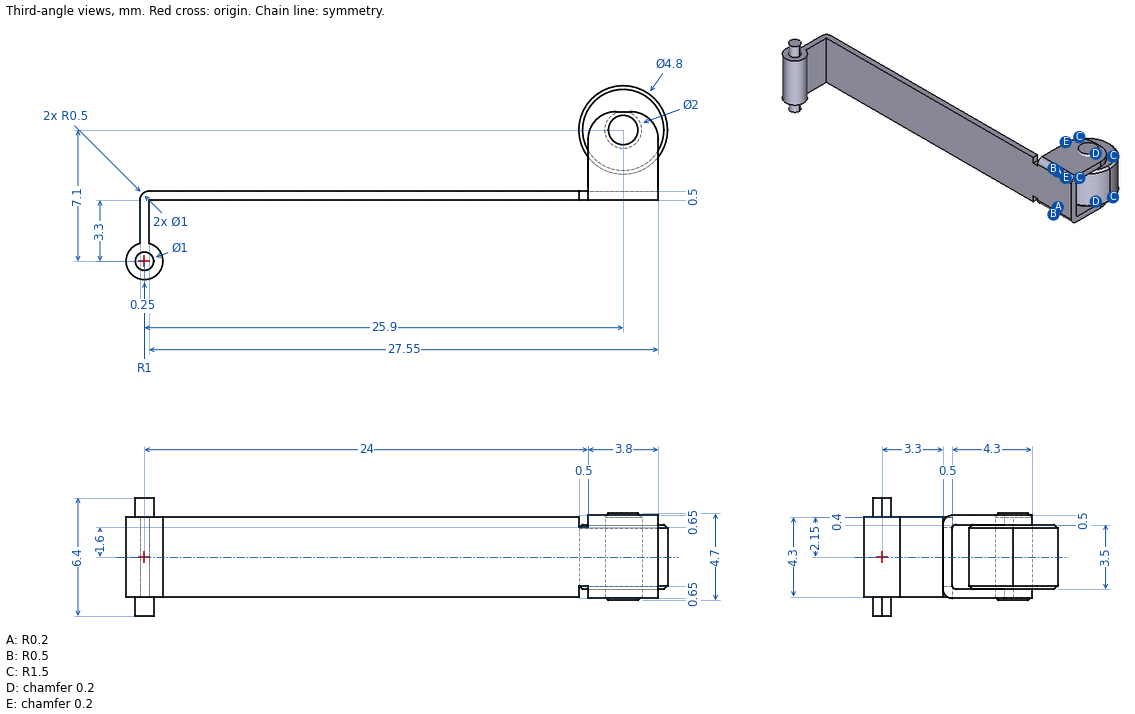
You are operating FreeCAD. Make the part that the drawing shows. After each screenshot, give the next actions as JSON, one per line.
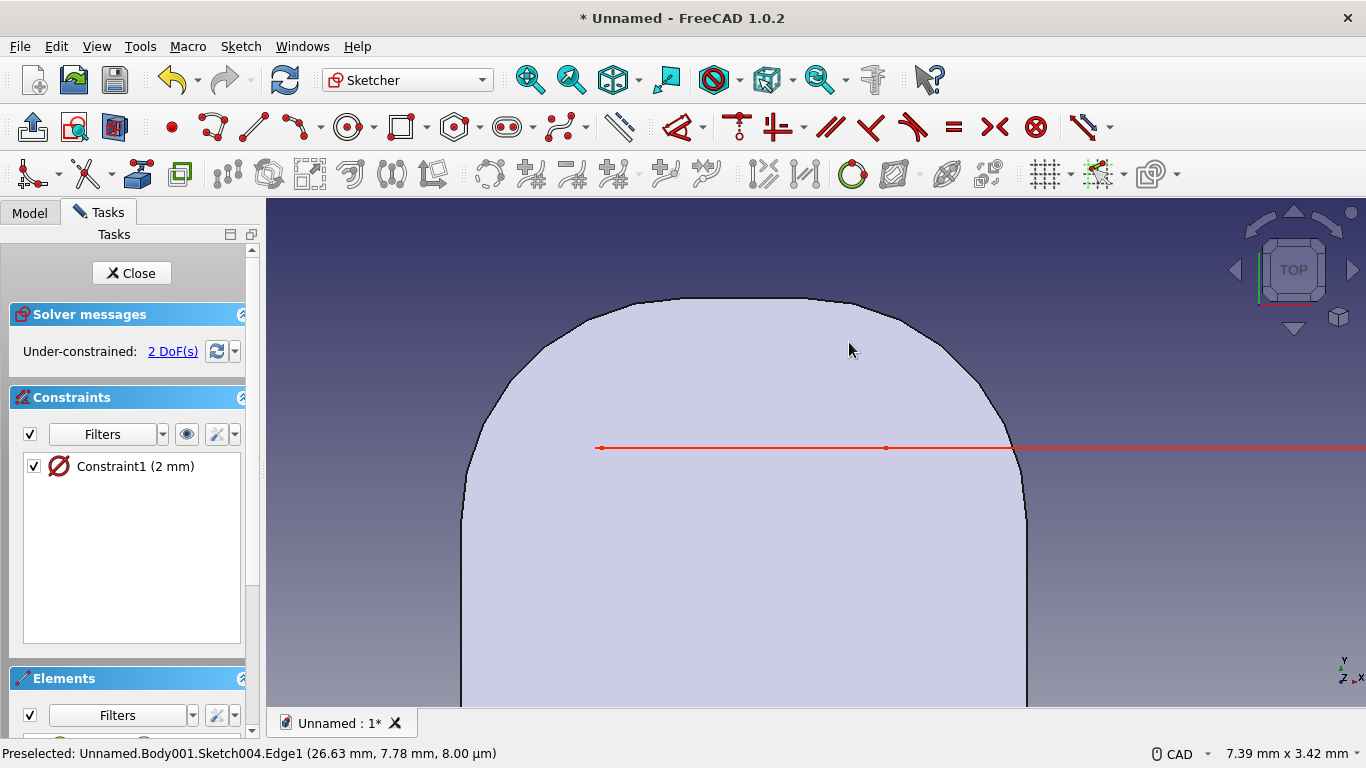
{"action": "key", "text": "d"}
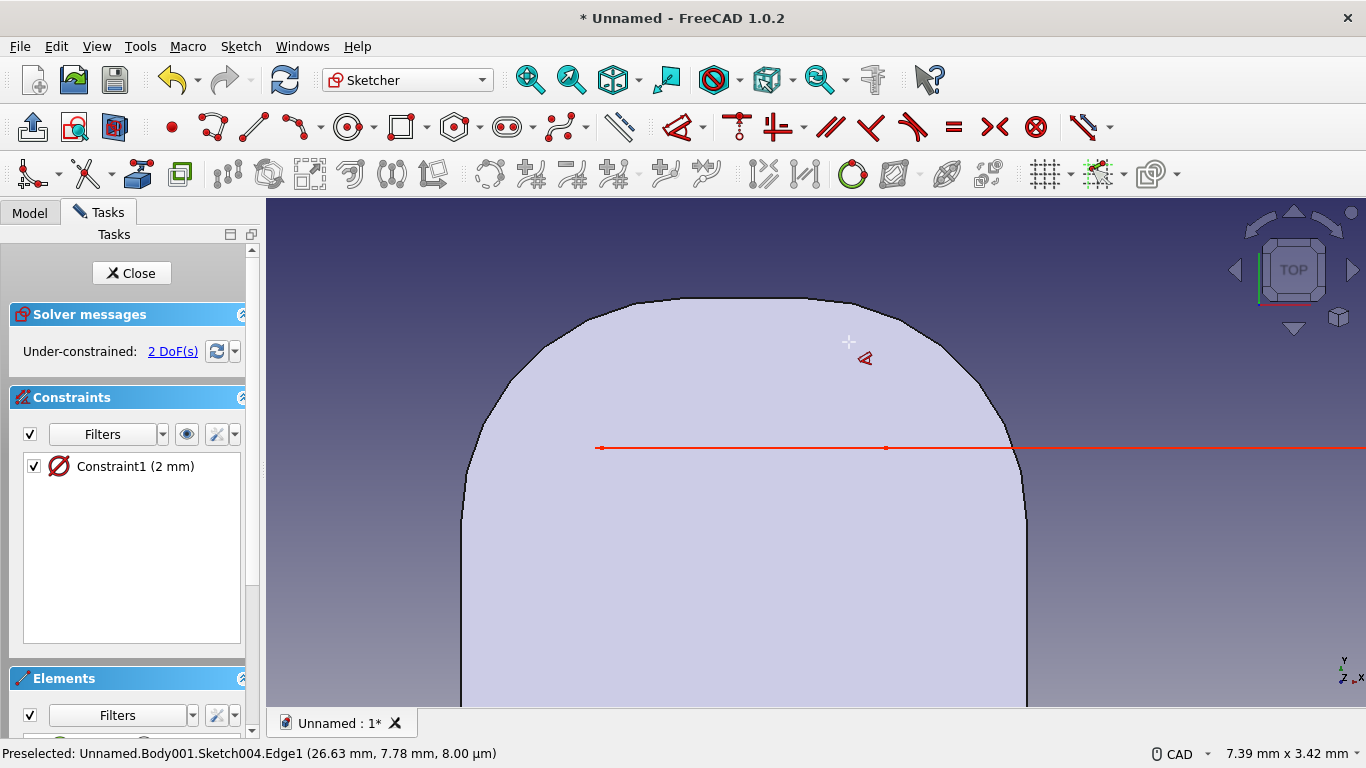
{"action": "left_click", "coordinate": [744, 448]}
{"action": "left_click", "coordinate": [778, 564]}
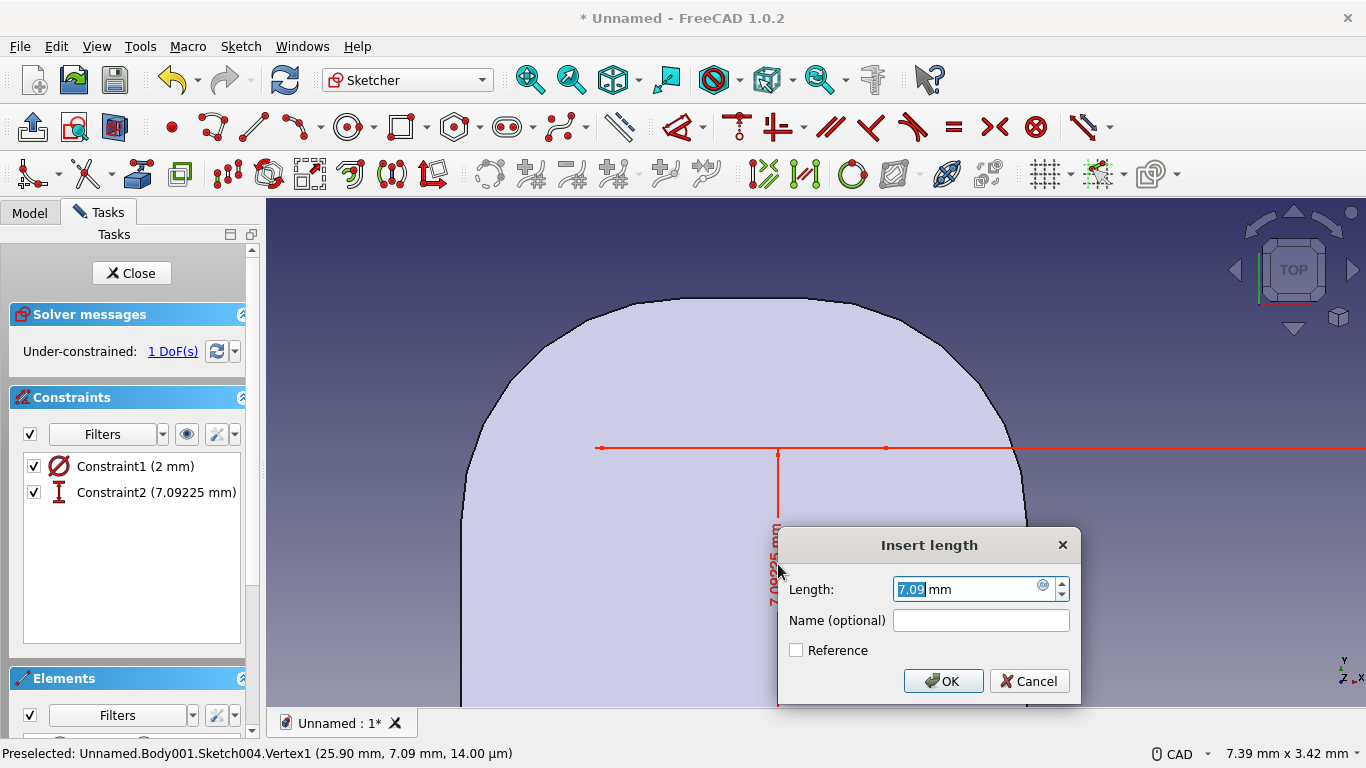
{"action": "type", "text": "7.1"}
{"action": "key", "text": "Return"}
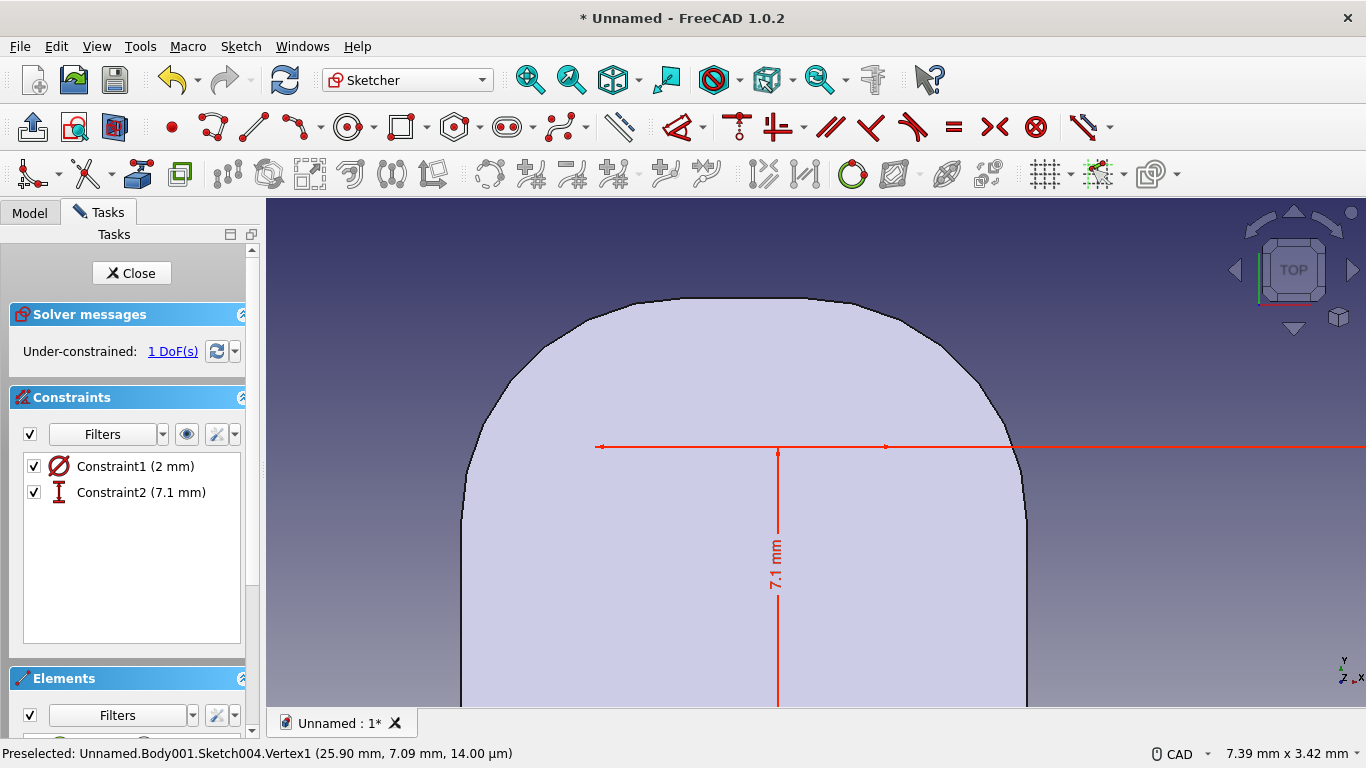
{"action": "left_click", "coordinate": [744, 447]}
{"action": "left_click", "coordinate": [519, 413]}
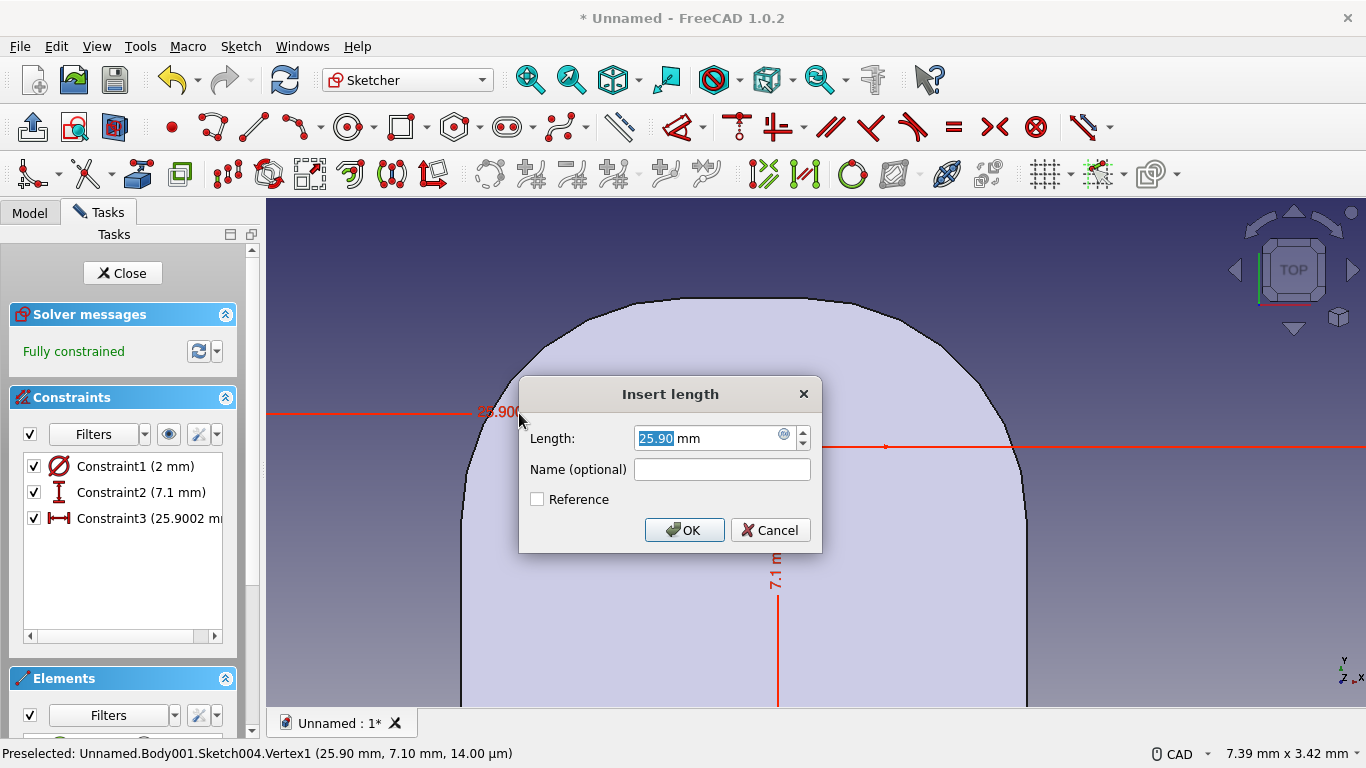
{"action": "type", "text": "25.9"}
{"action": "key", "text": "Return"}
{"action": "key", "text": "Escape"}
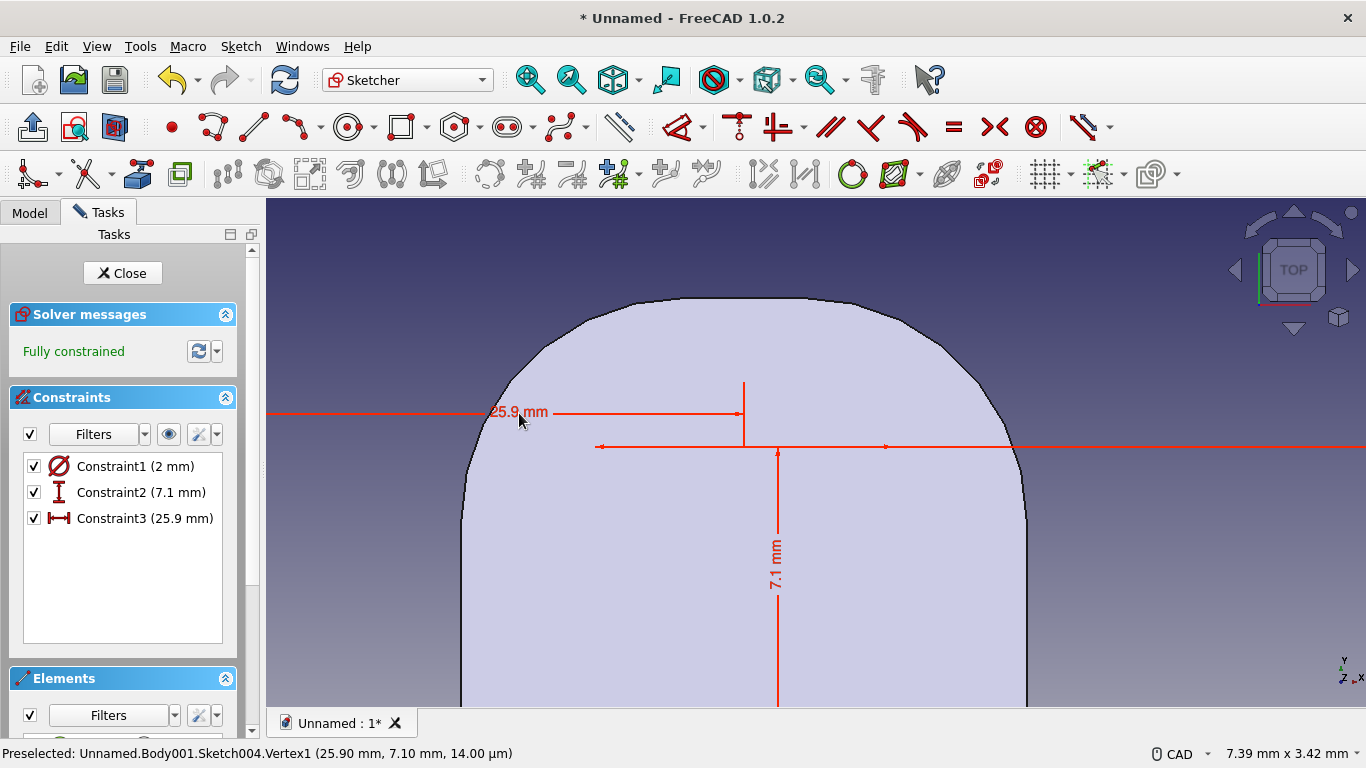
{"action": "left_click", "coordinate": [123, 273]}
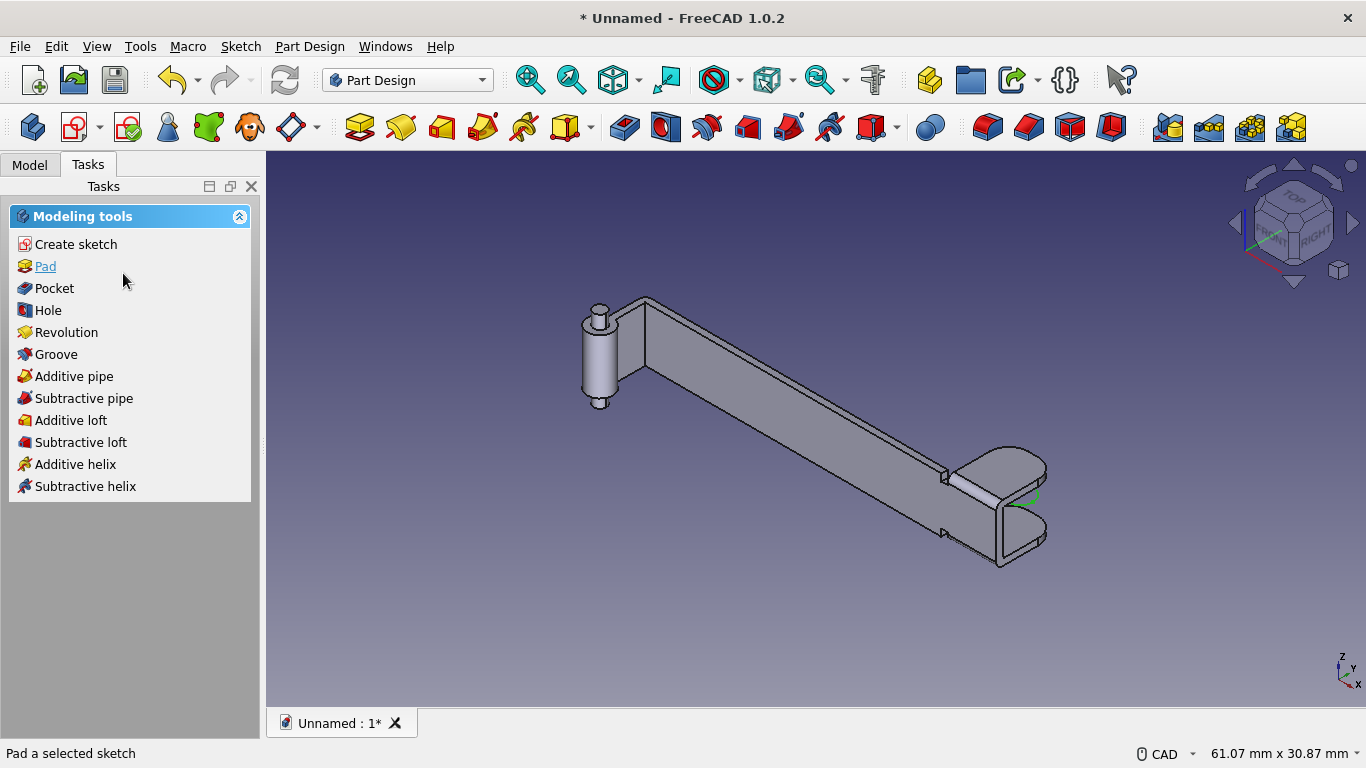
{"action": "left_click", "coordinate": [360, 128]}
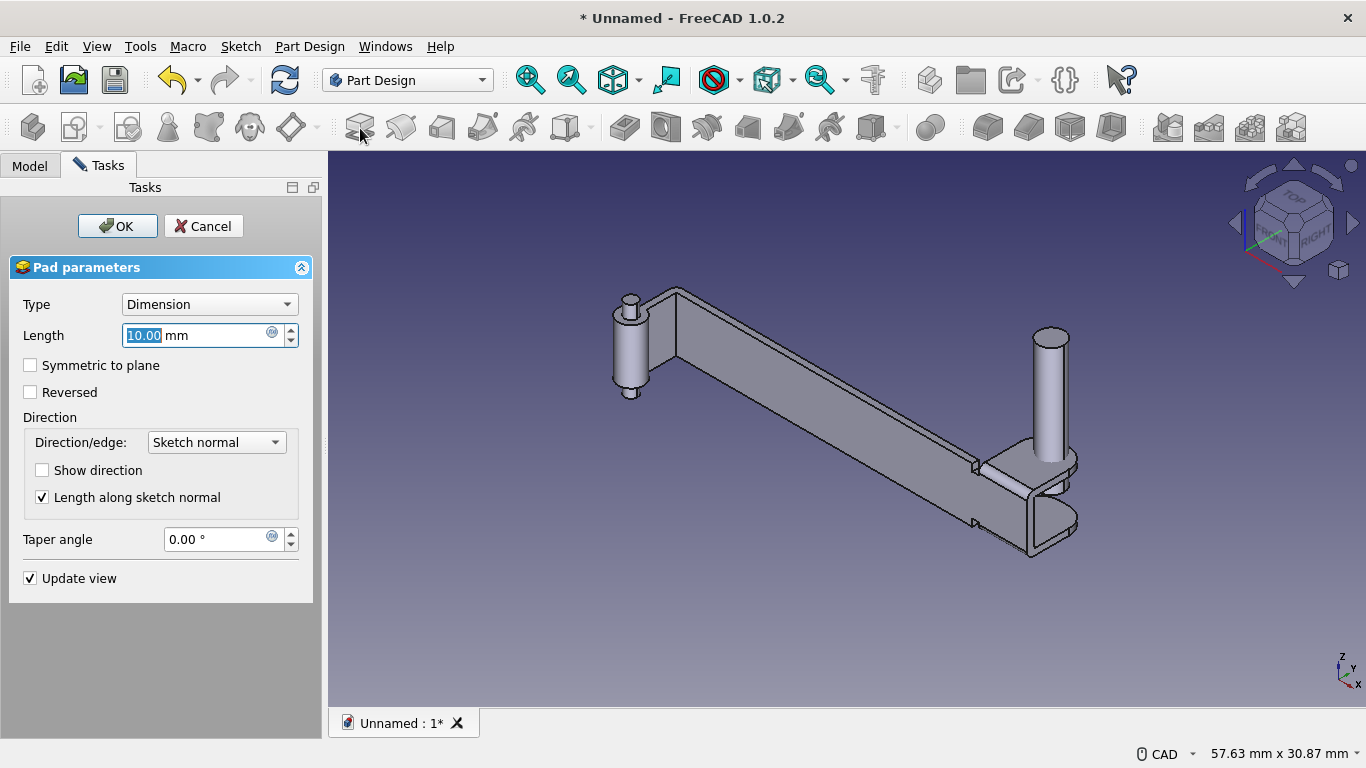
{"action": "type", "text": "4.7"}
{"action": "key", "text": "Tab"}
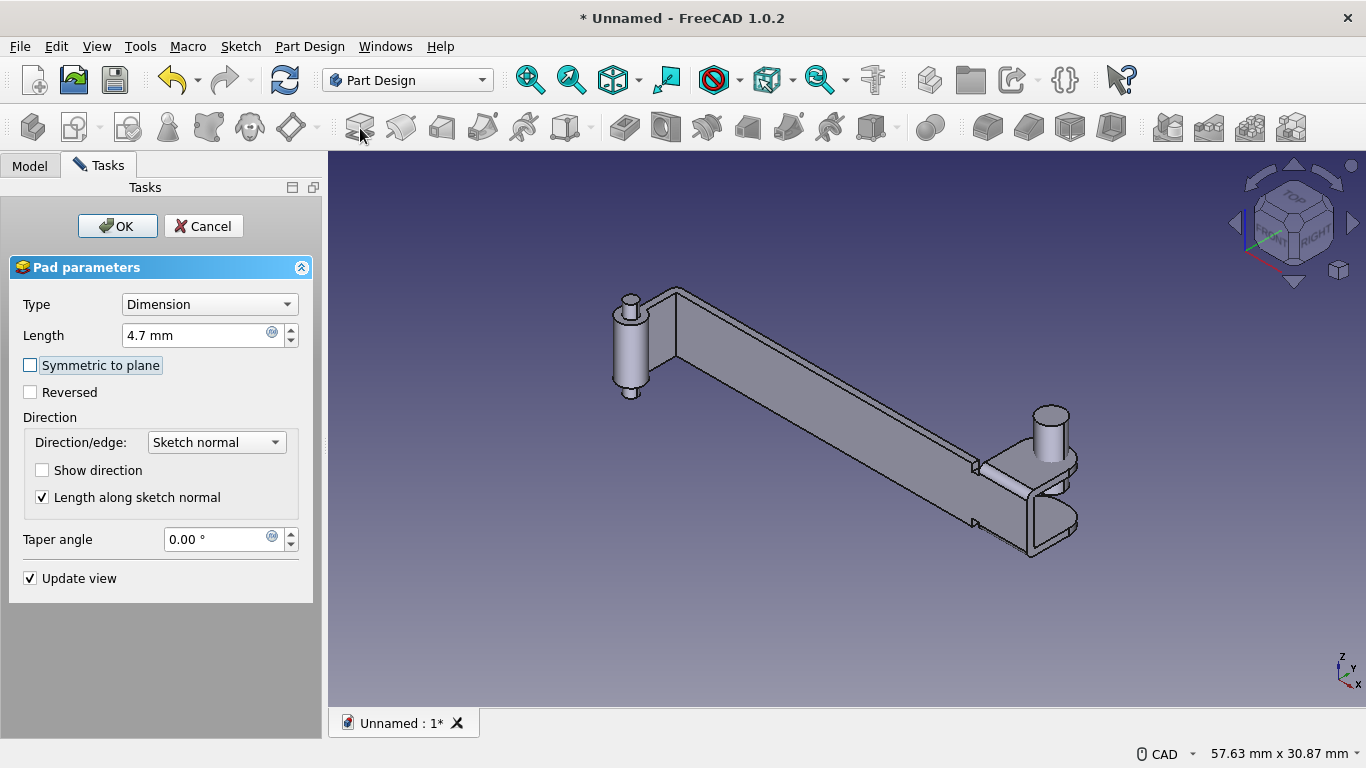
{"action": "left_click", "coordinate": [31, 365]}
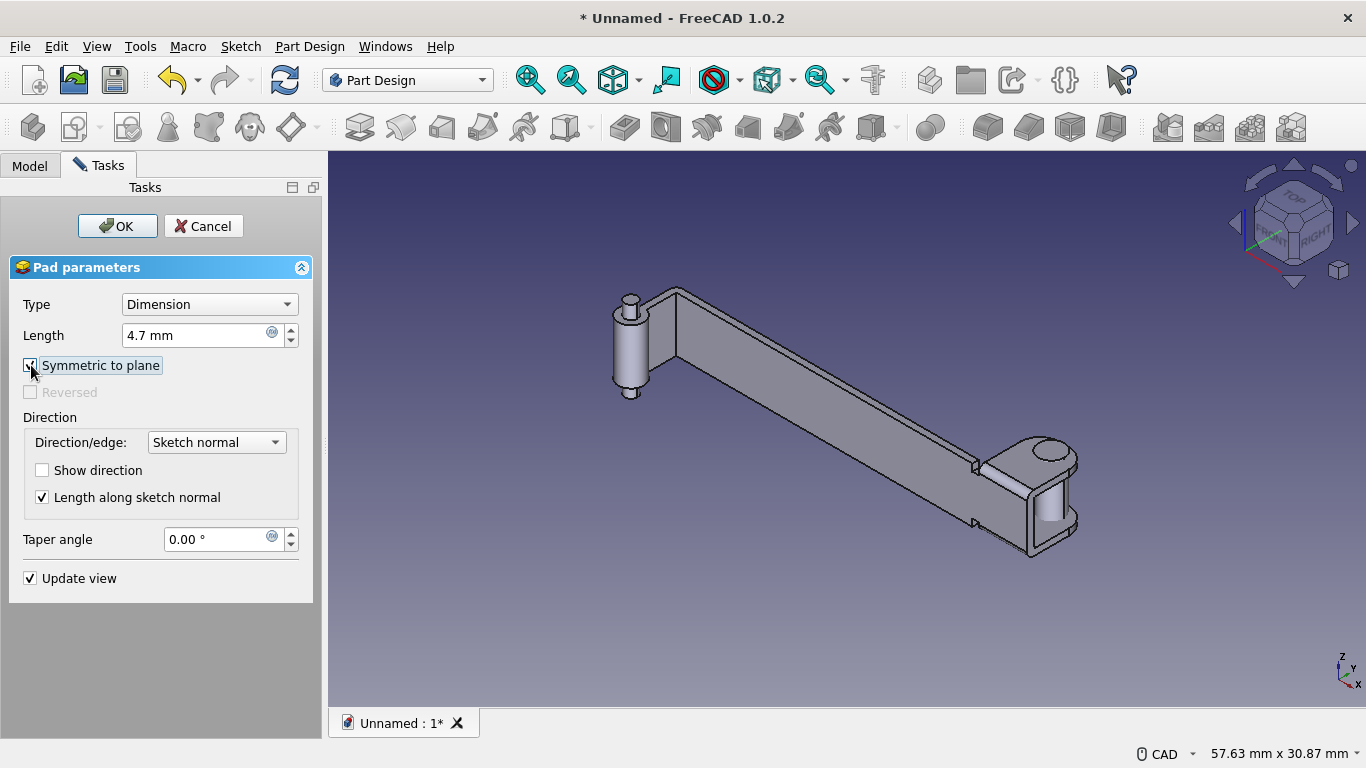
{"action": "left_click", "coordinate": [118, 226]}